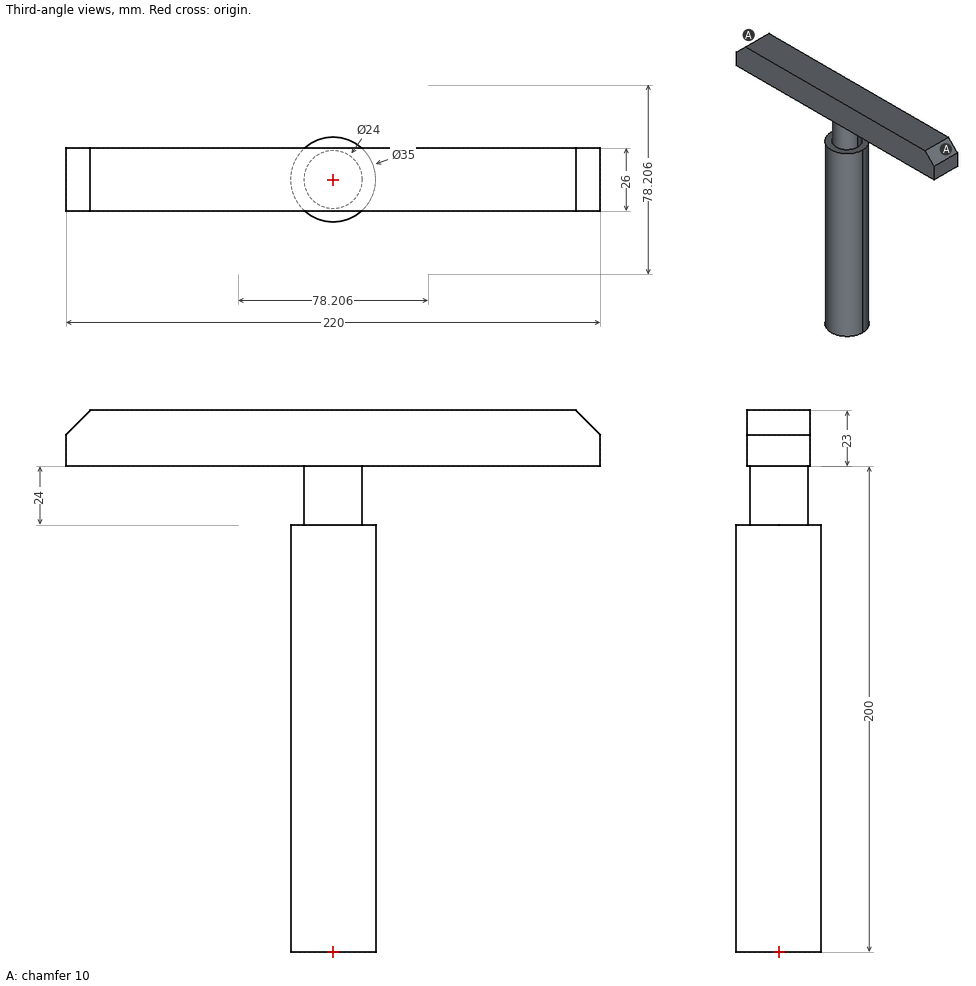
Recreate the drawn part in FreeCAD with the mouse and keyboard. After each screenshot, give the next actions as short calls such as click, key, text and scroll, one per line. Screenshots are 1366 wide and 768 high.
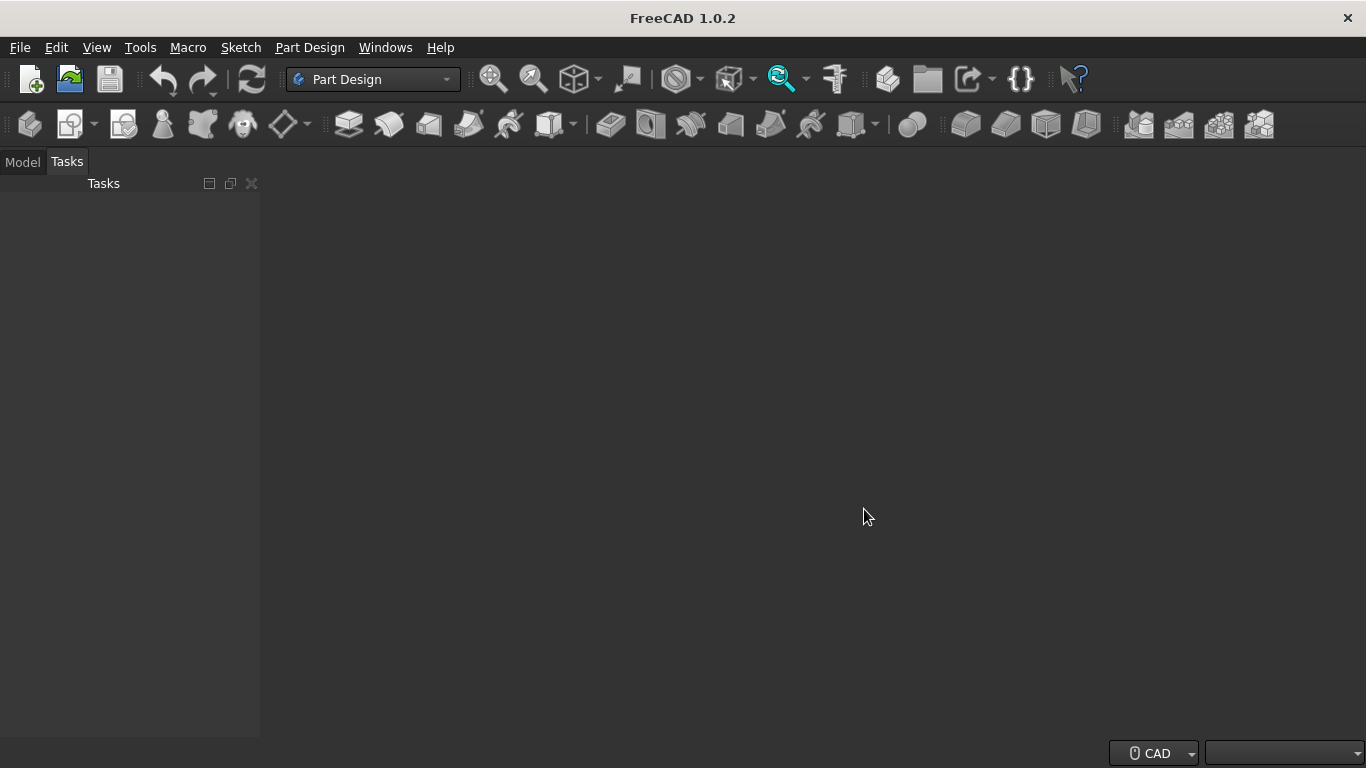
click(30, 80)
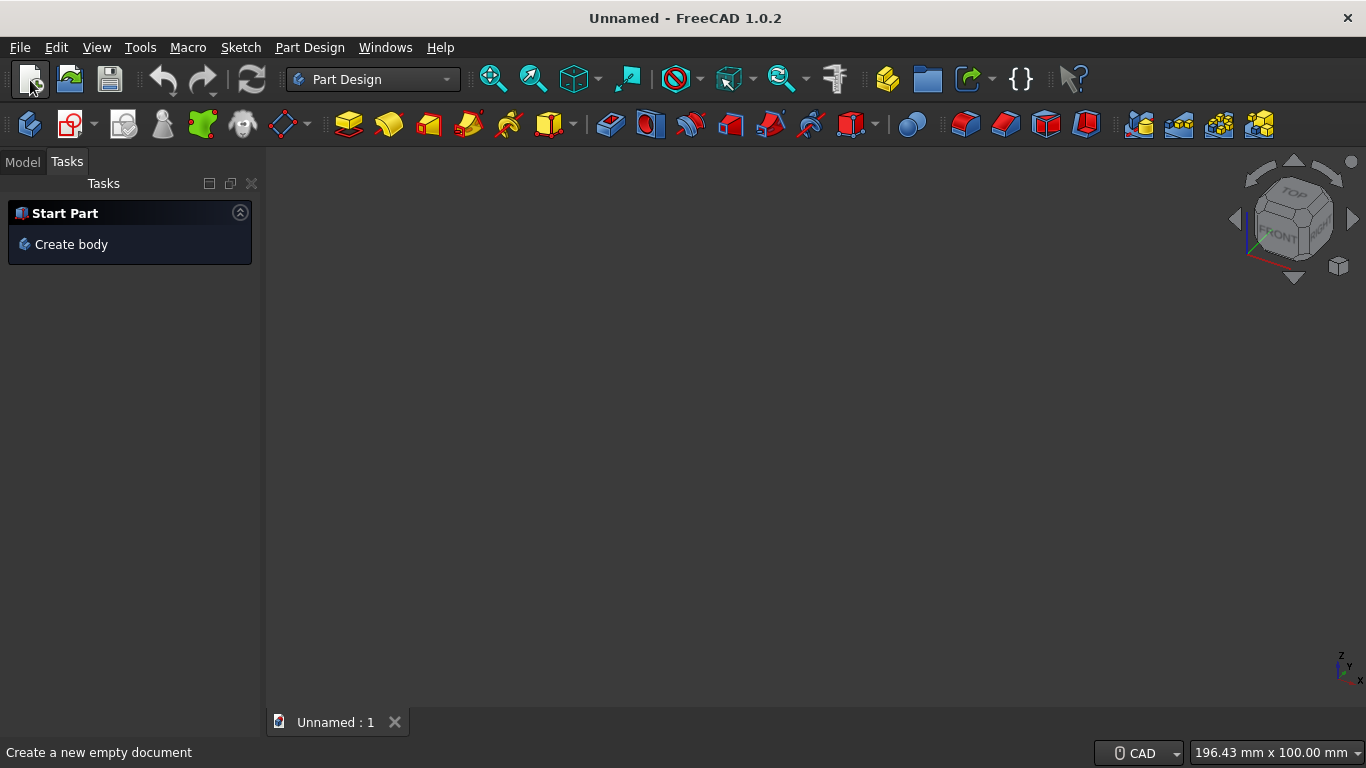
click(70, 124)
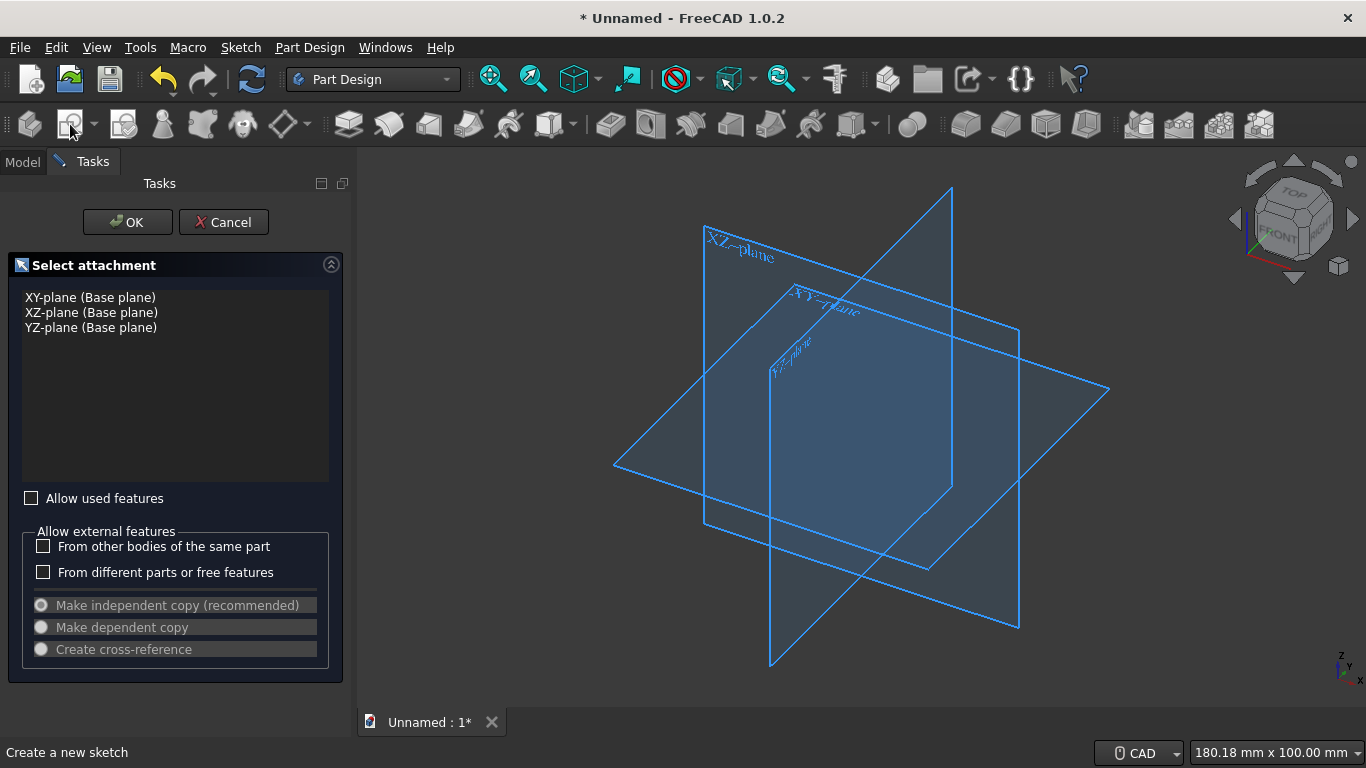
click(82, 298)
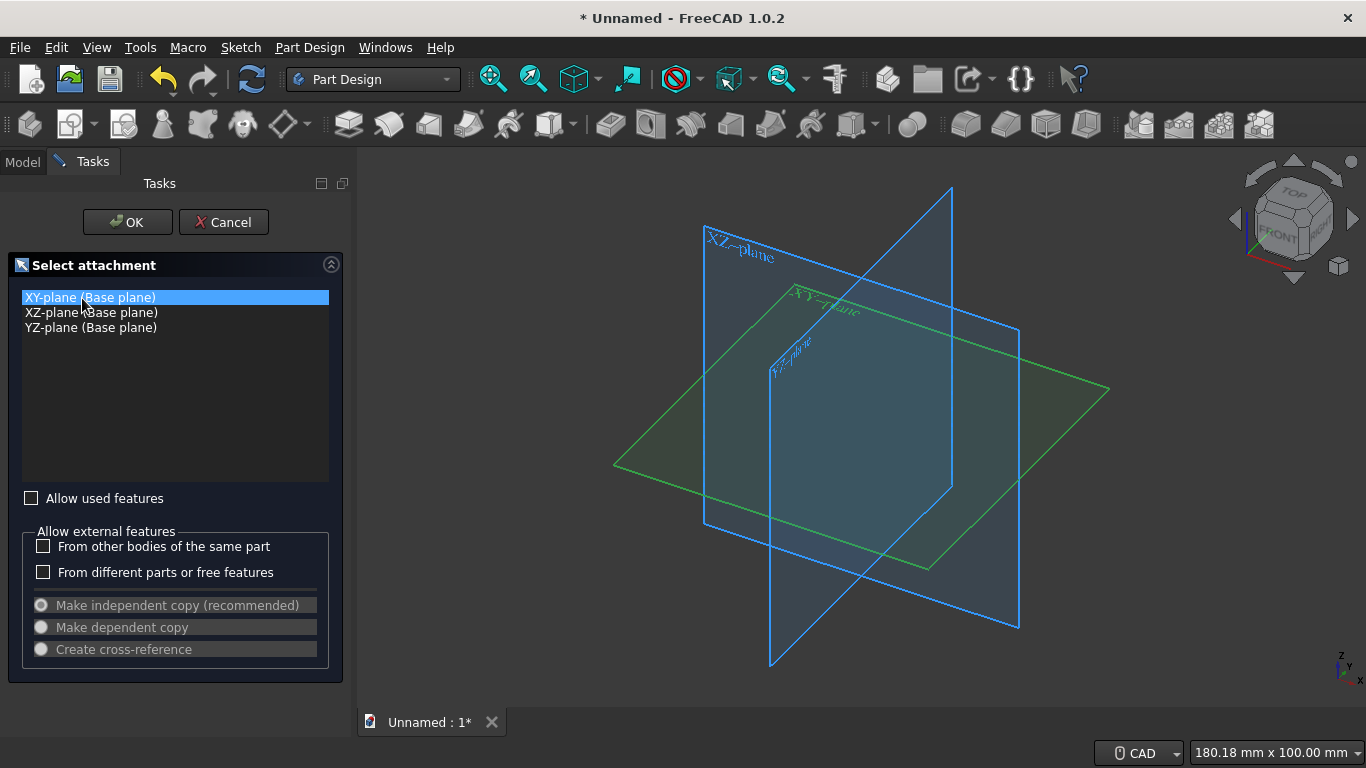
click(128, 222)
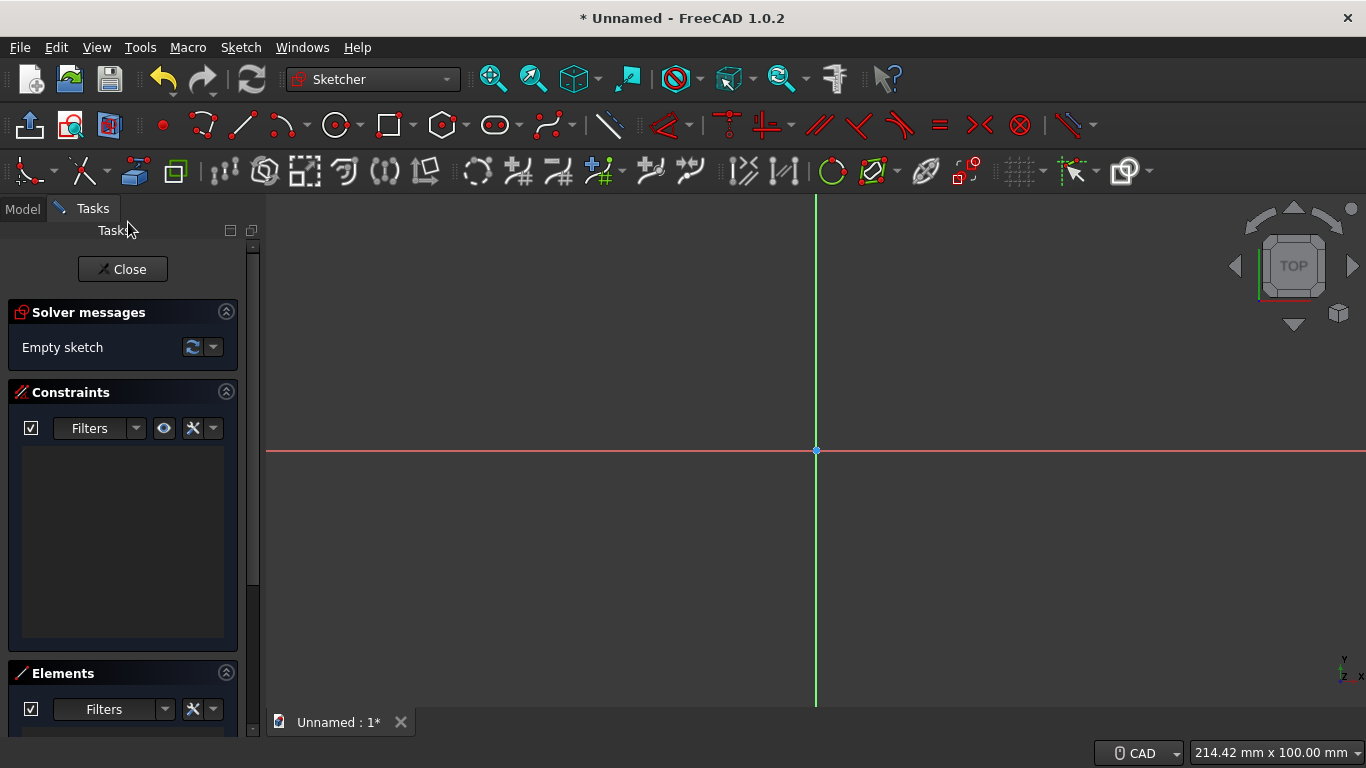
scroll(899, 450, up, 3)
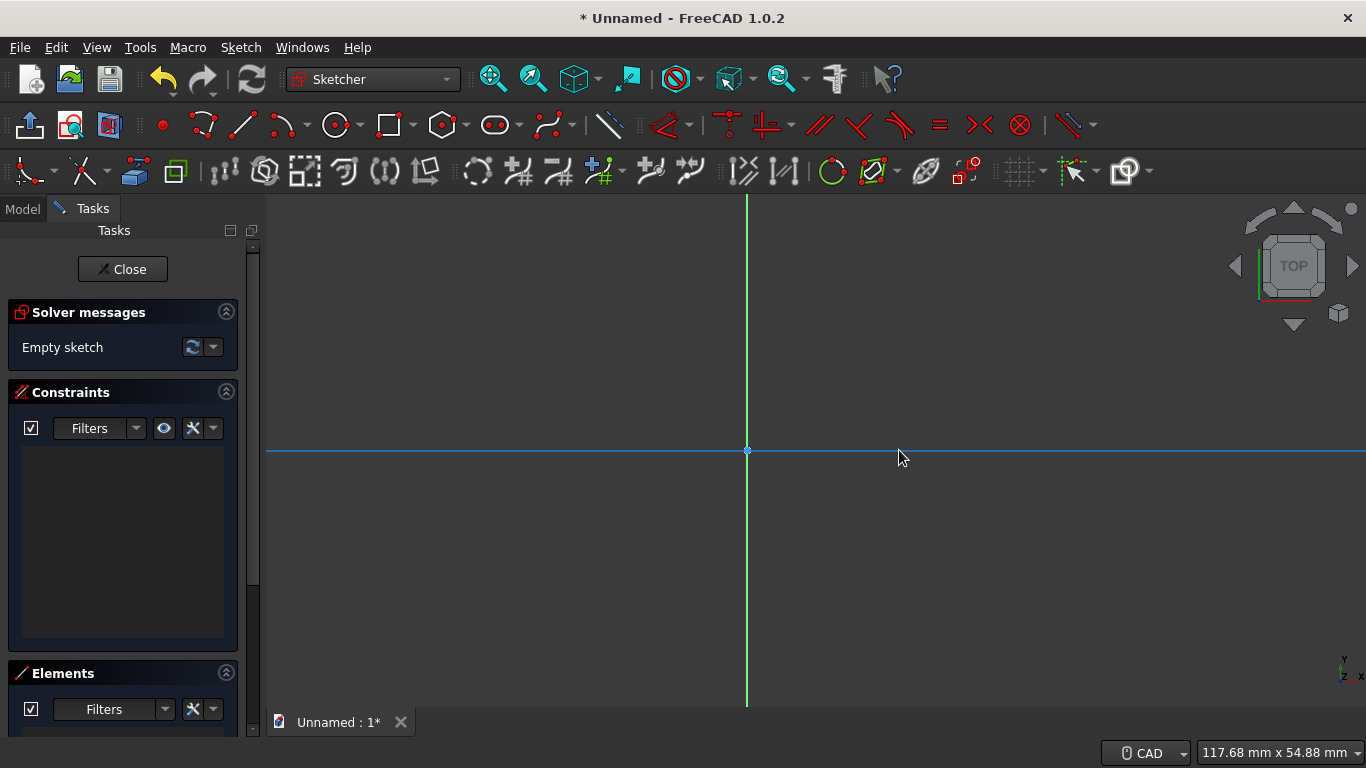
key(g)
key(c)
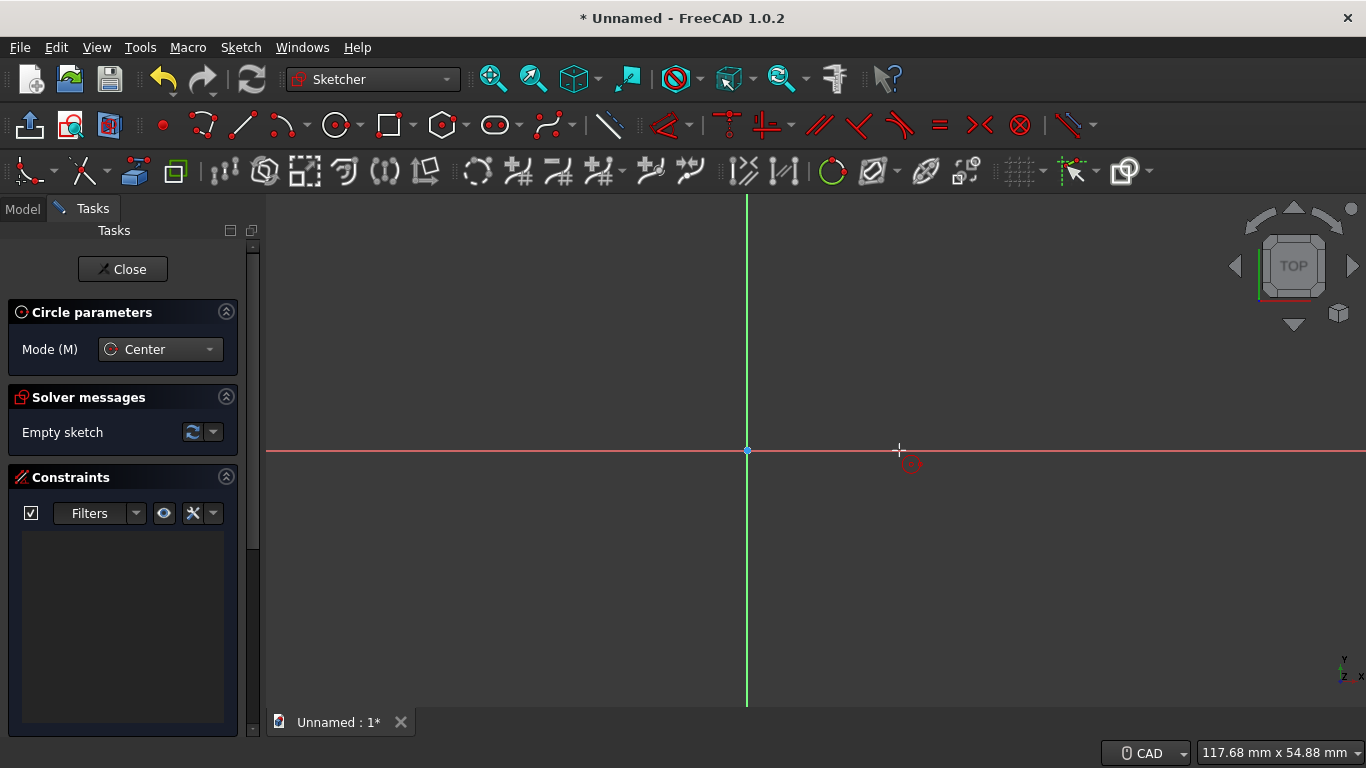
click(747, 450)
click(863, 335)
key(Escape)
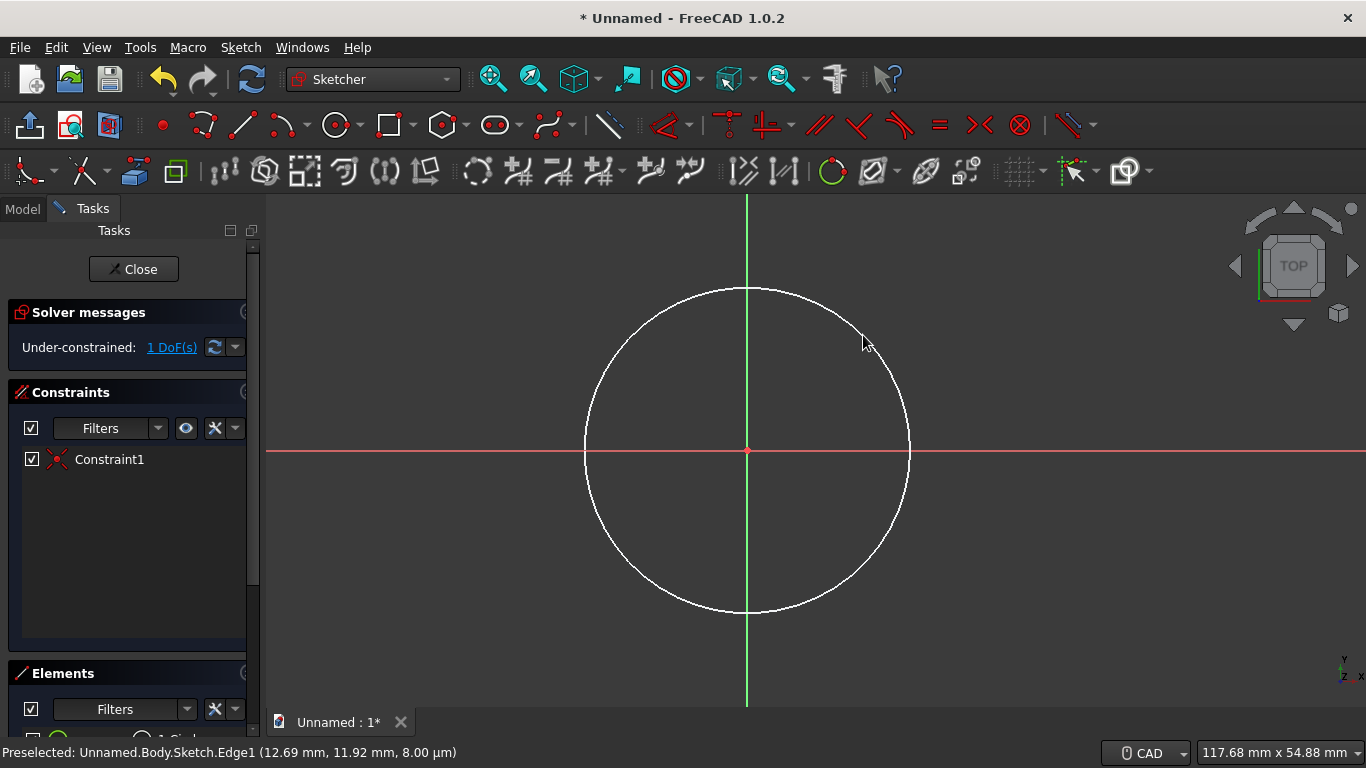
click(664, 126)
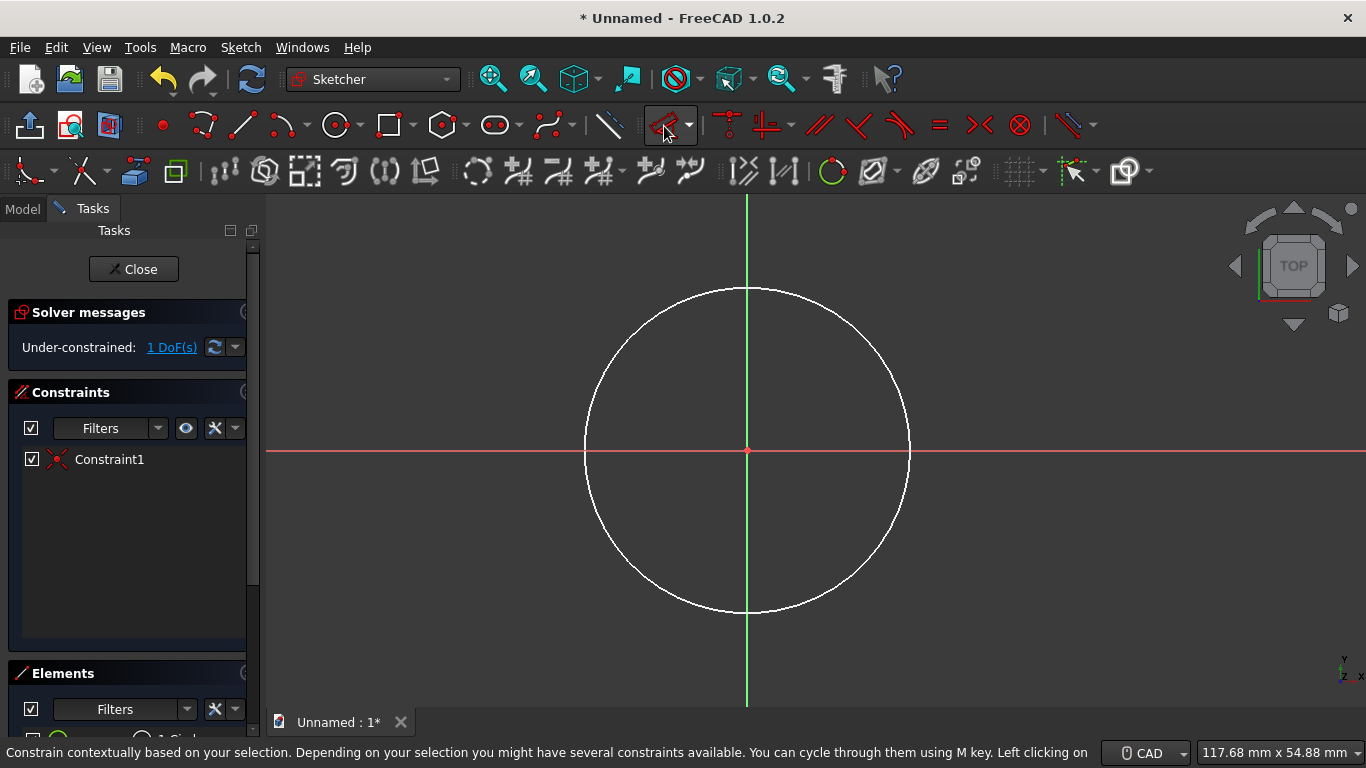
click(862, 335)
click(885, 312)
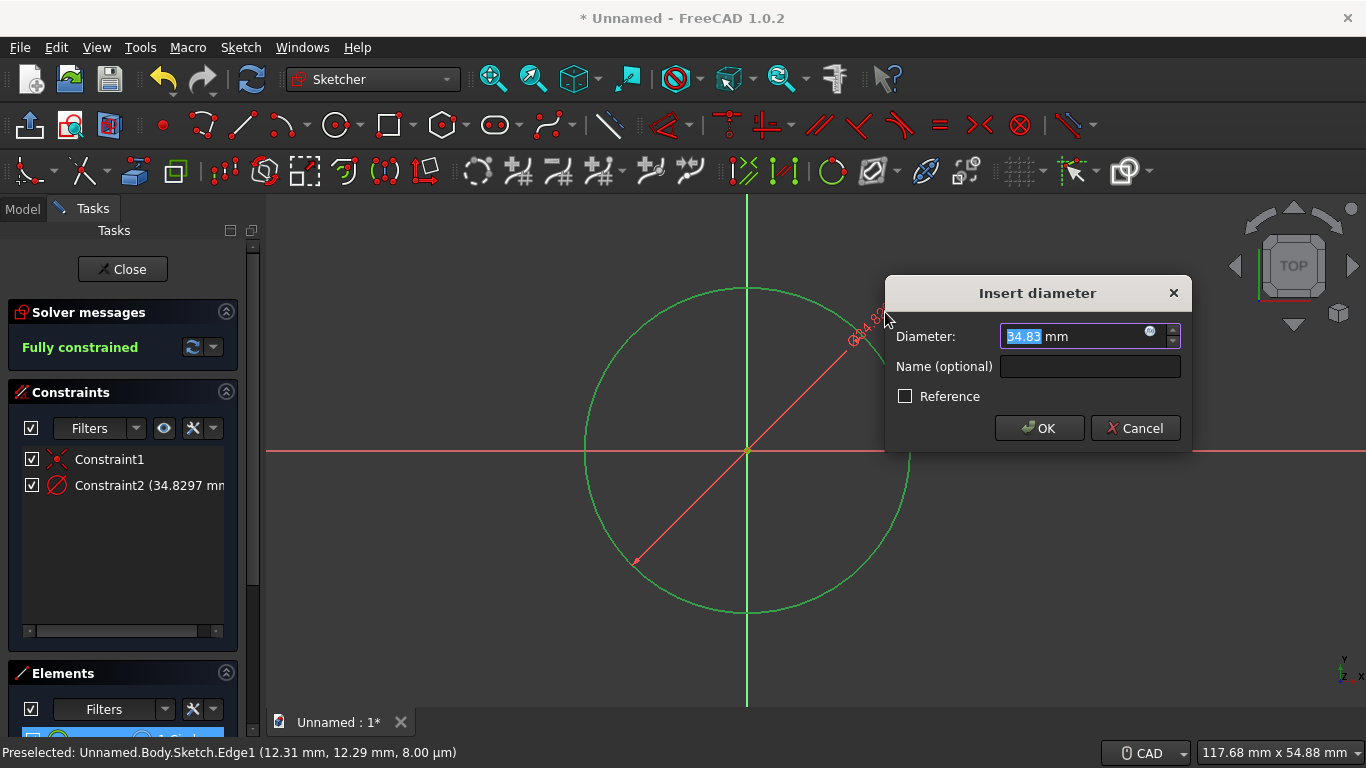
text(35)
key(Return)
key(Escape)